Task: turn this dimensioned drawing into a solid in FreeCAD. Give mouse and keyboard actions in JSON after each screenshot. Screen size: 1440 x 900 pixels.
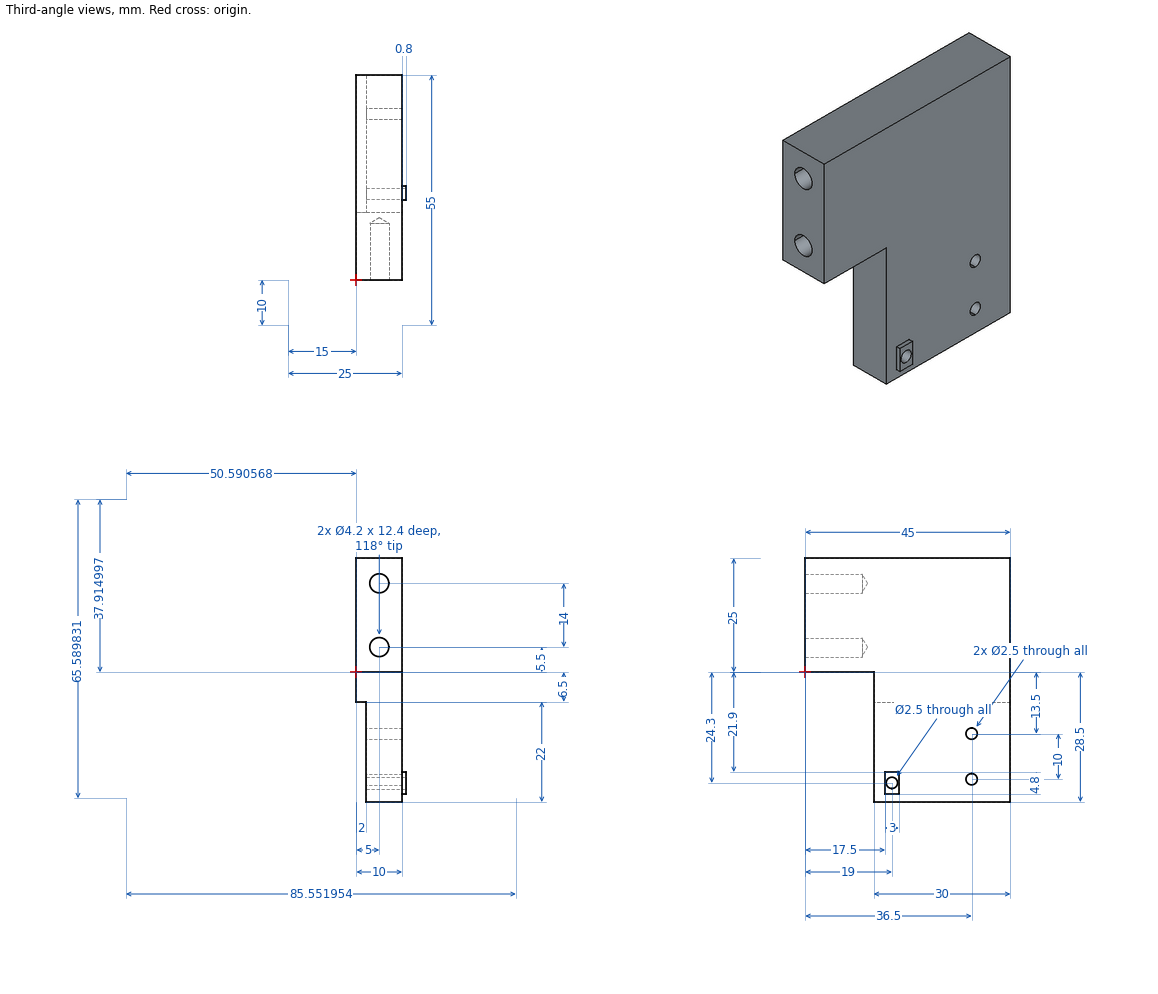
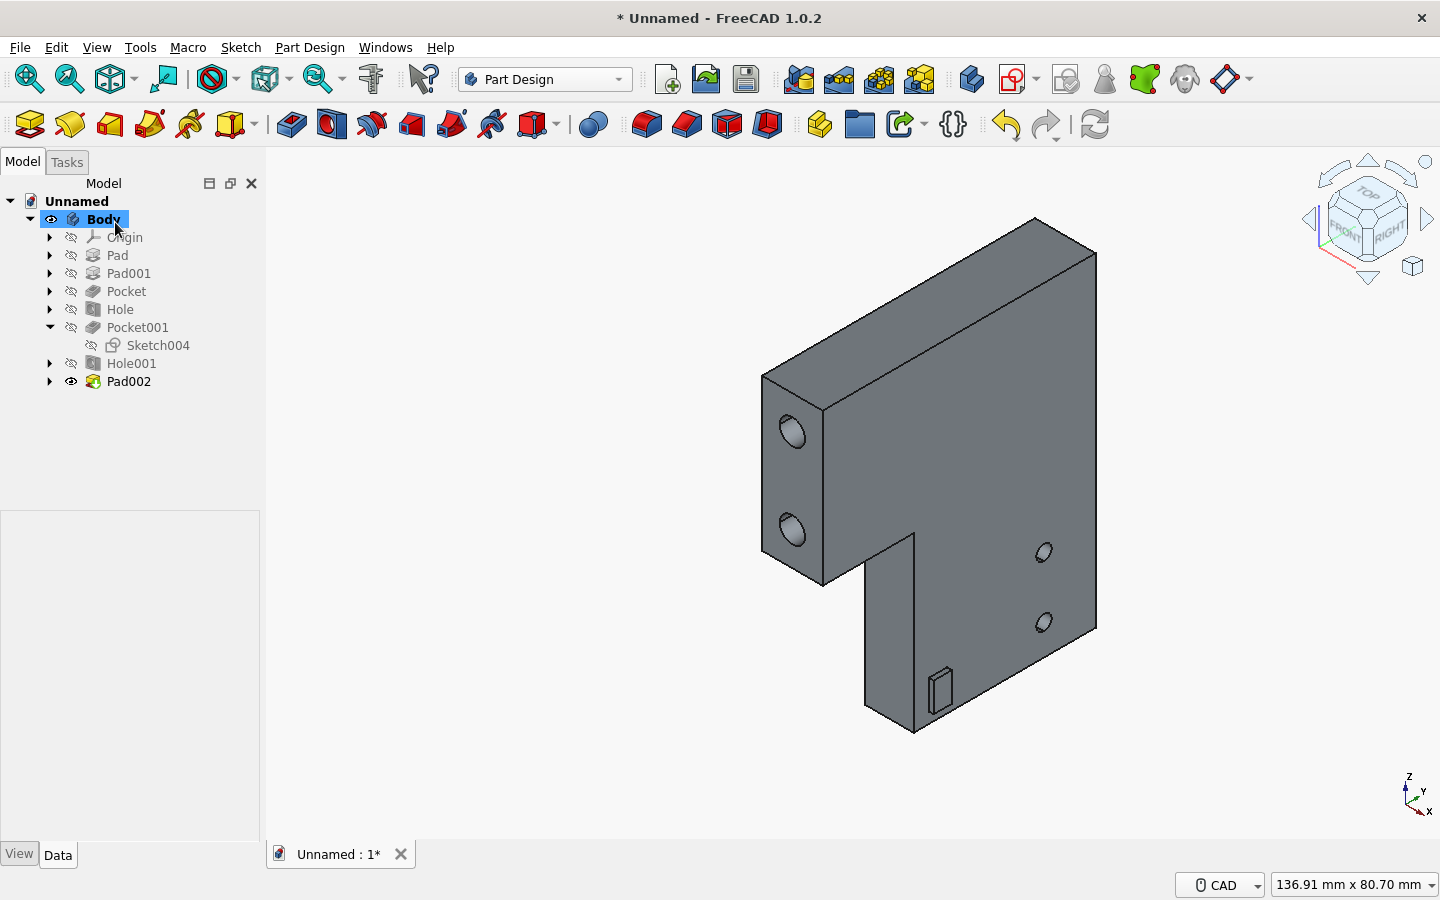
{"action": "left_click", "coordinate": [1012, 80]}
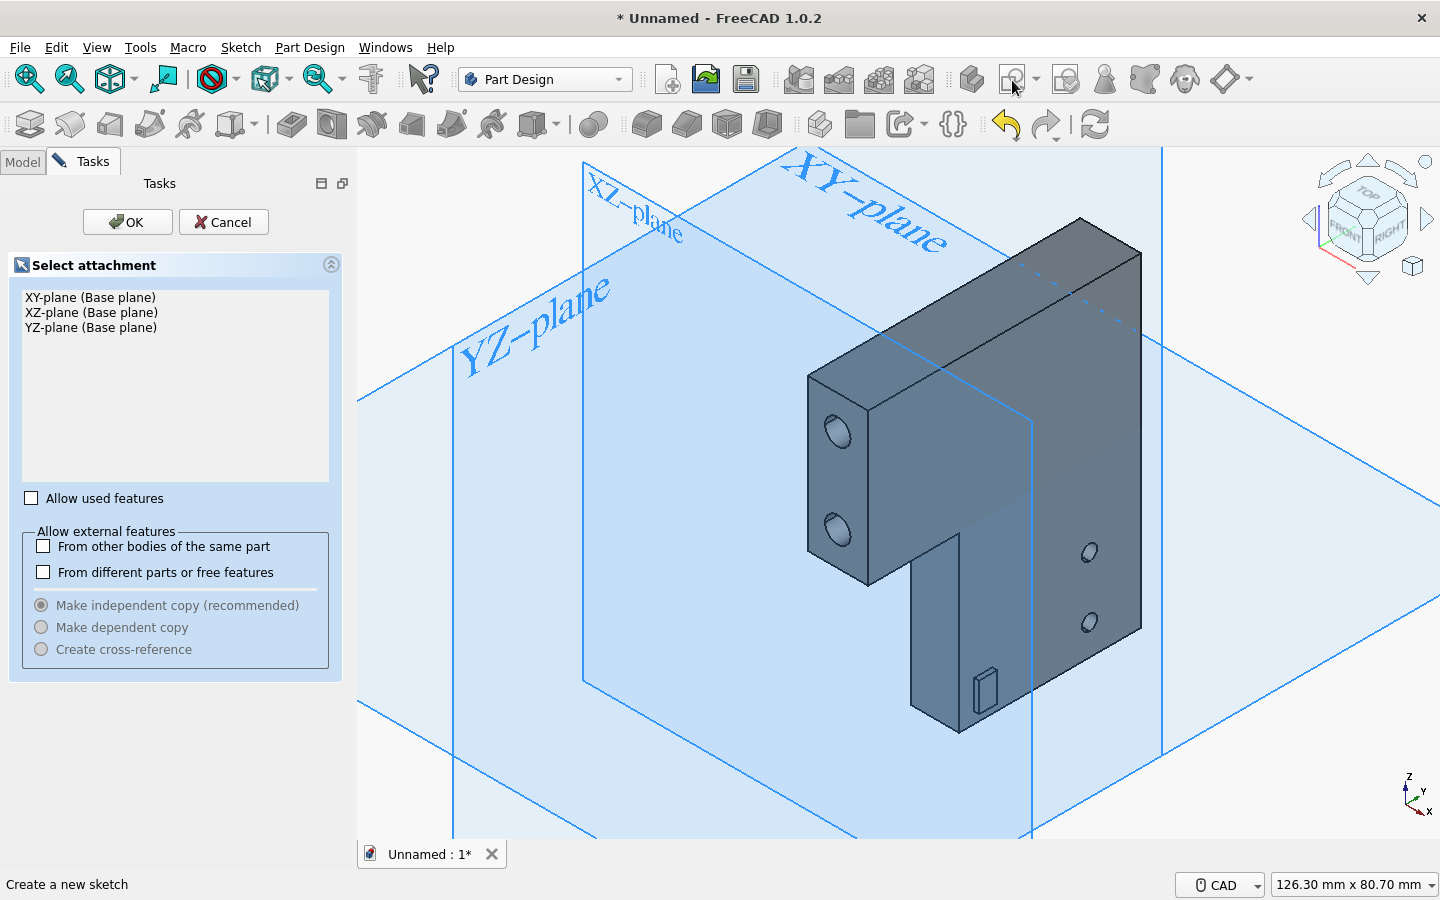
{"action": "left_click", "coordinate": [82, 328]}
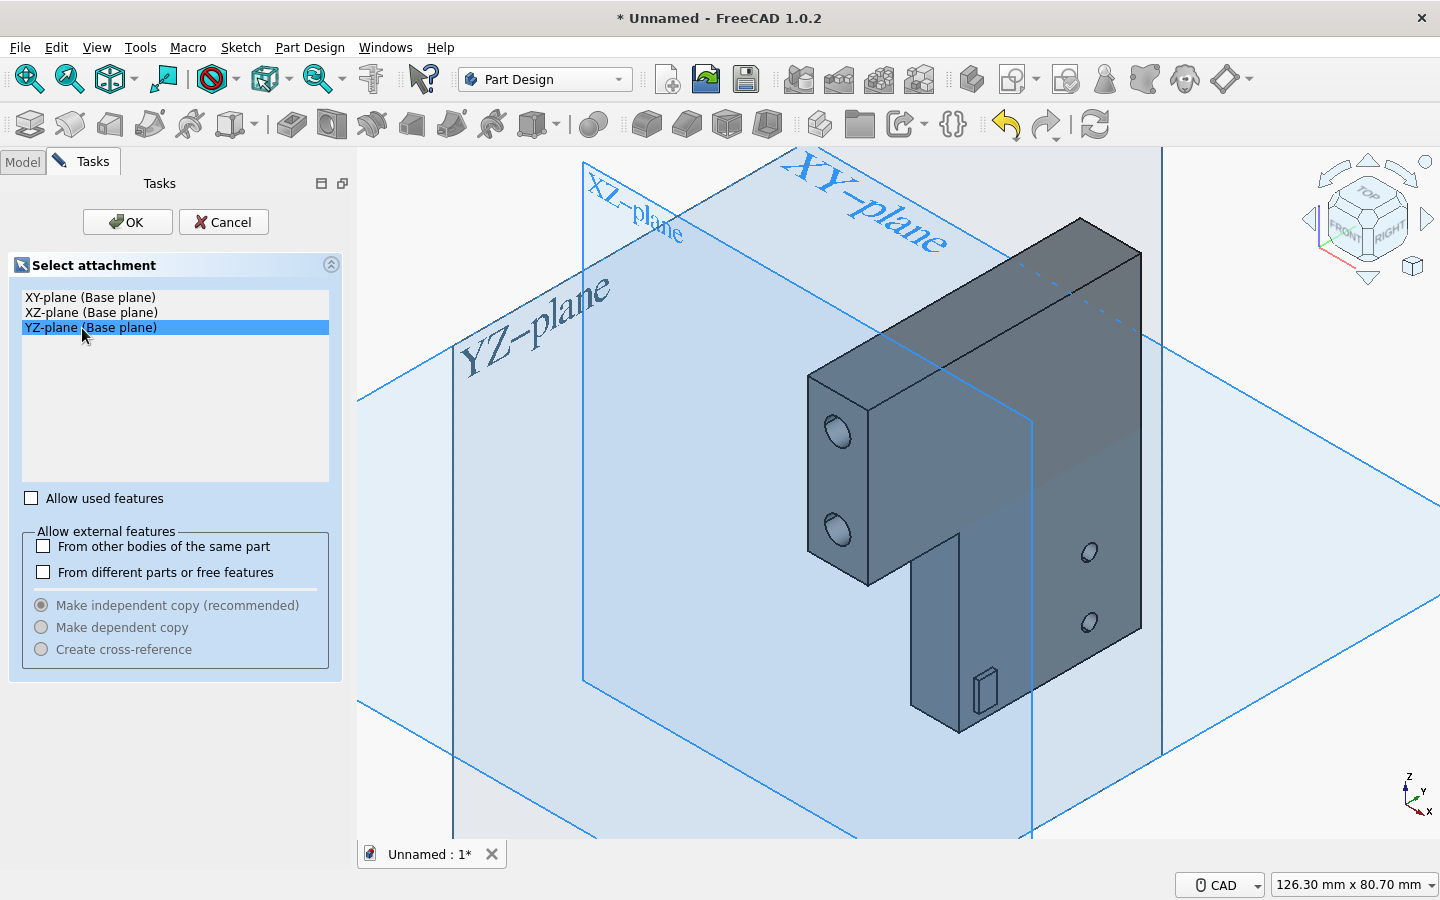
{"action": "left_click", "coordinate": [128, 222]}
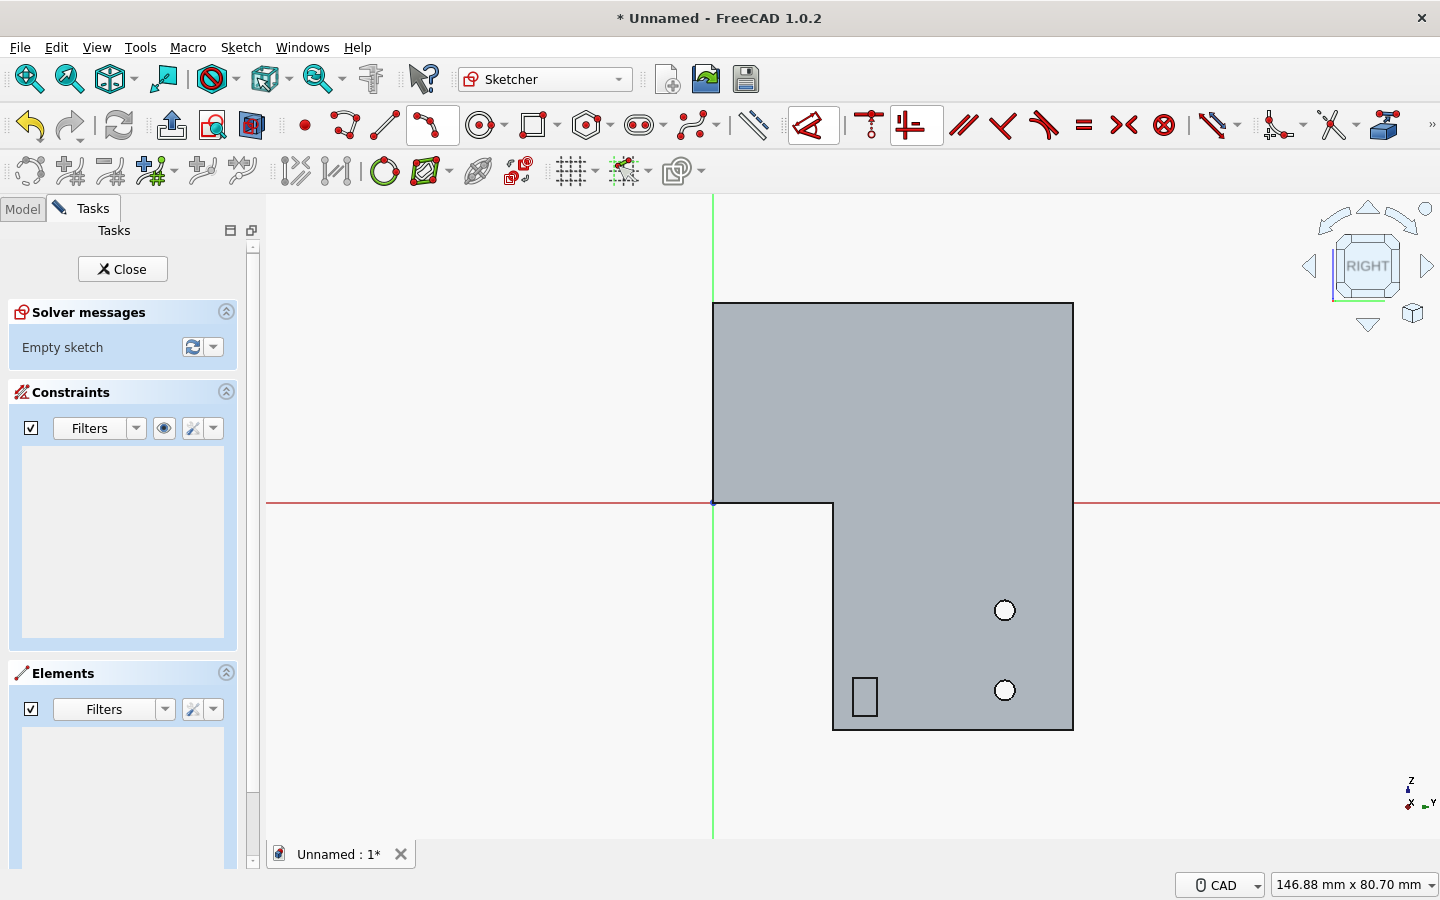
{"action": "left_click", "coordinate": [252, 126]}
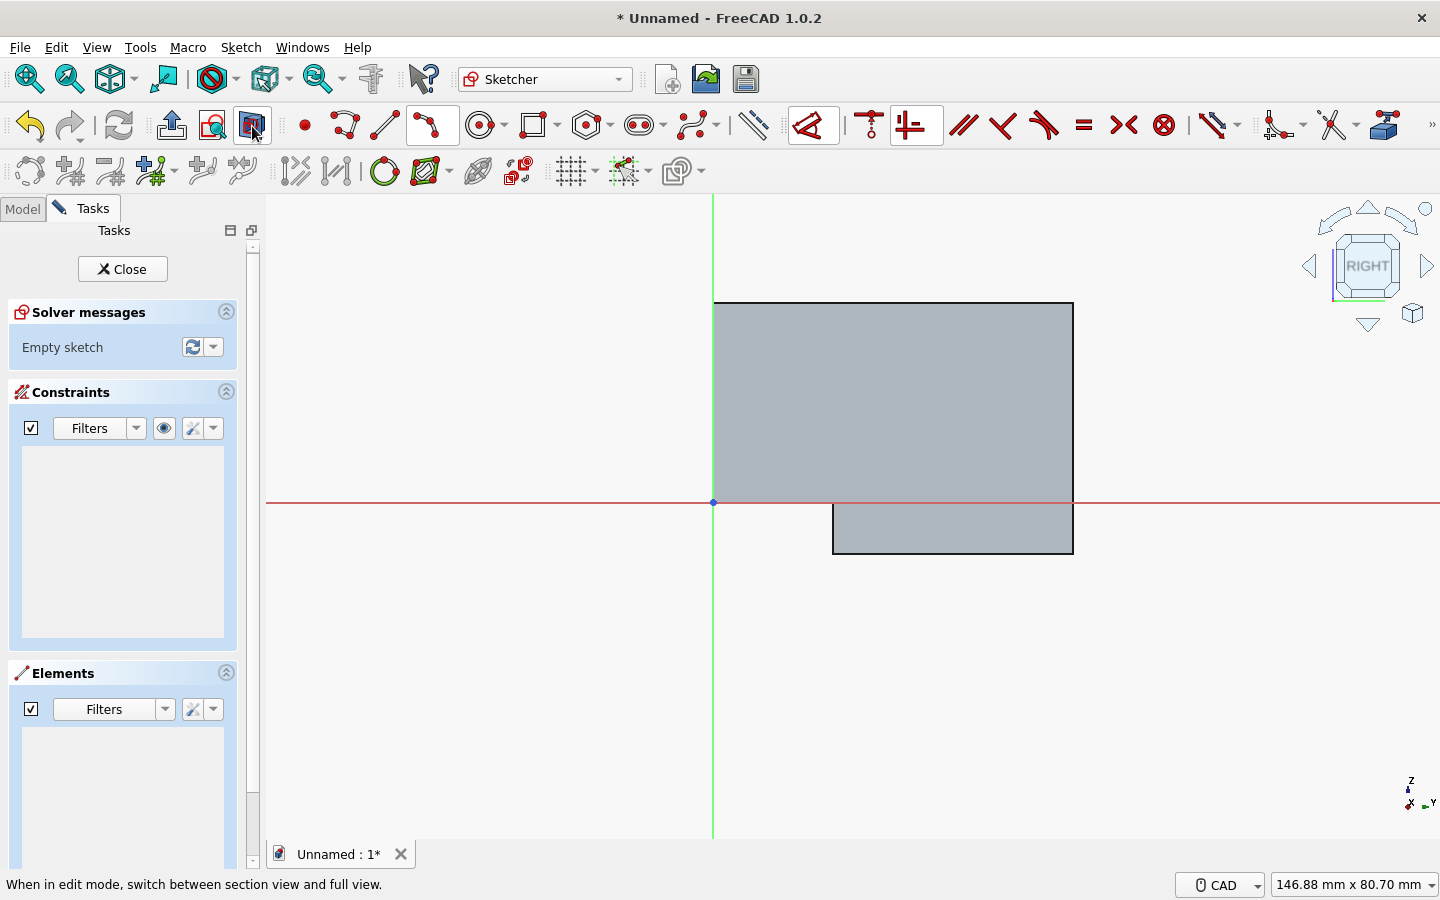
{"action": "scroll", "coordinate": [869, 706], "scroll_direction": "up", "scroll_amount": 15}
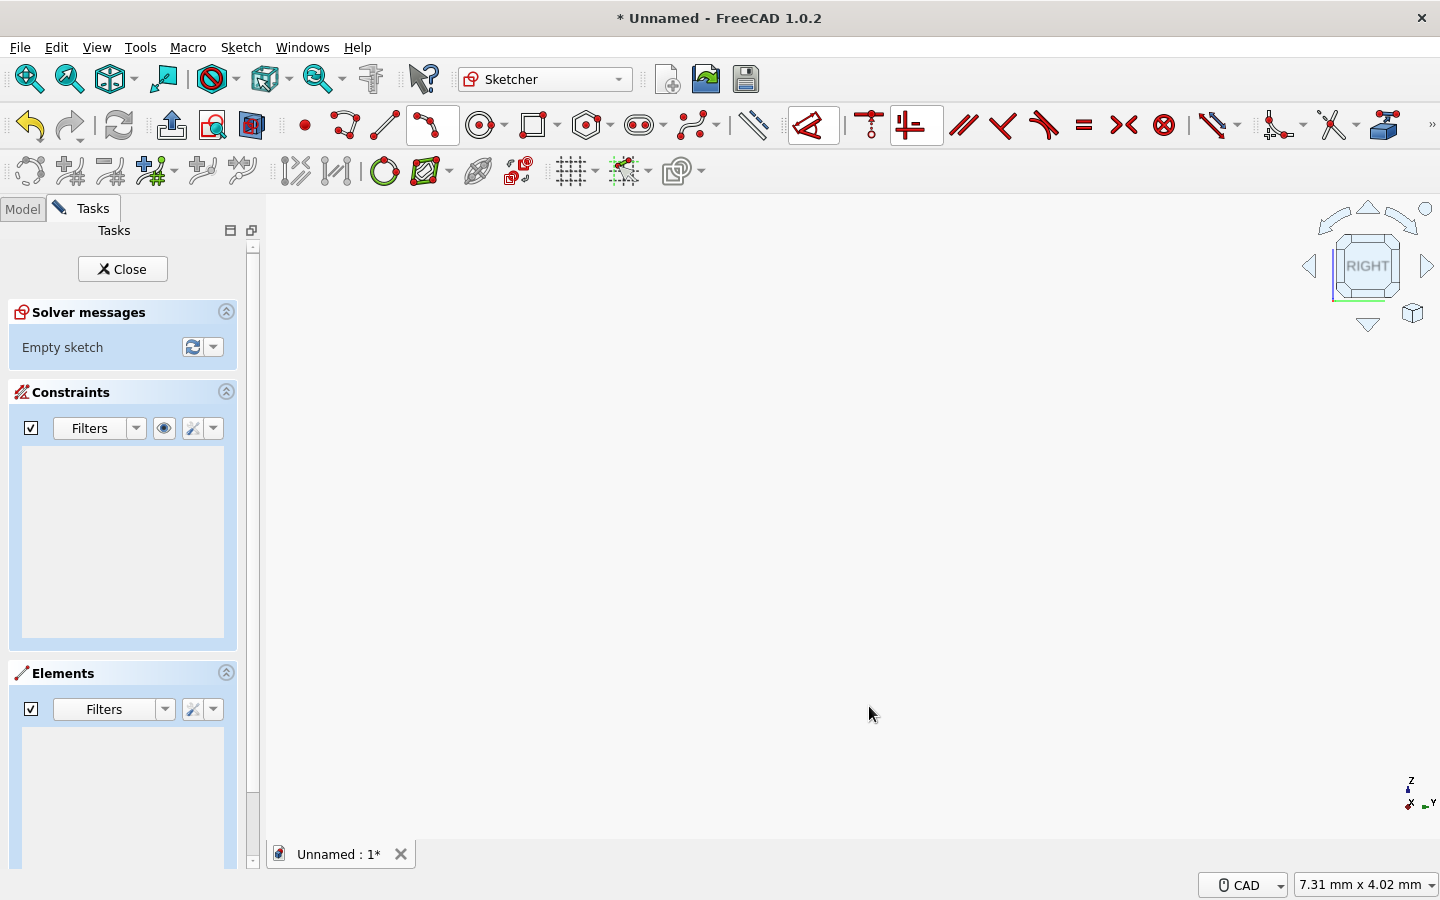
{"action": "left_click", "coordinate": [480, 126]}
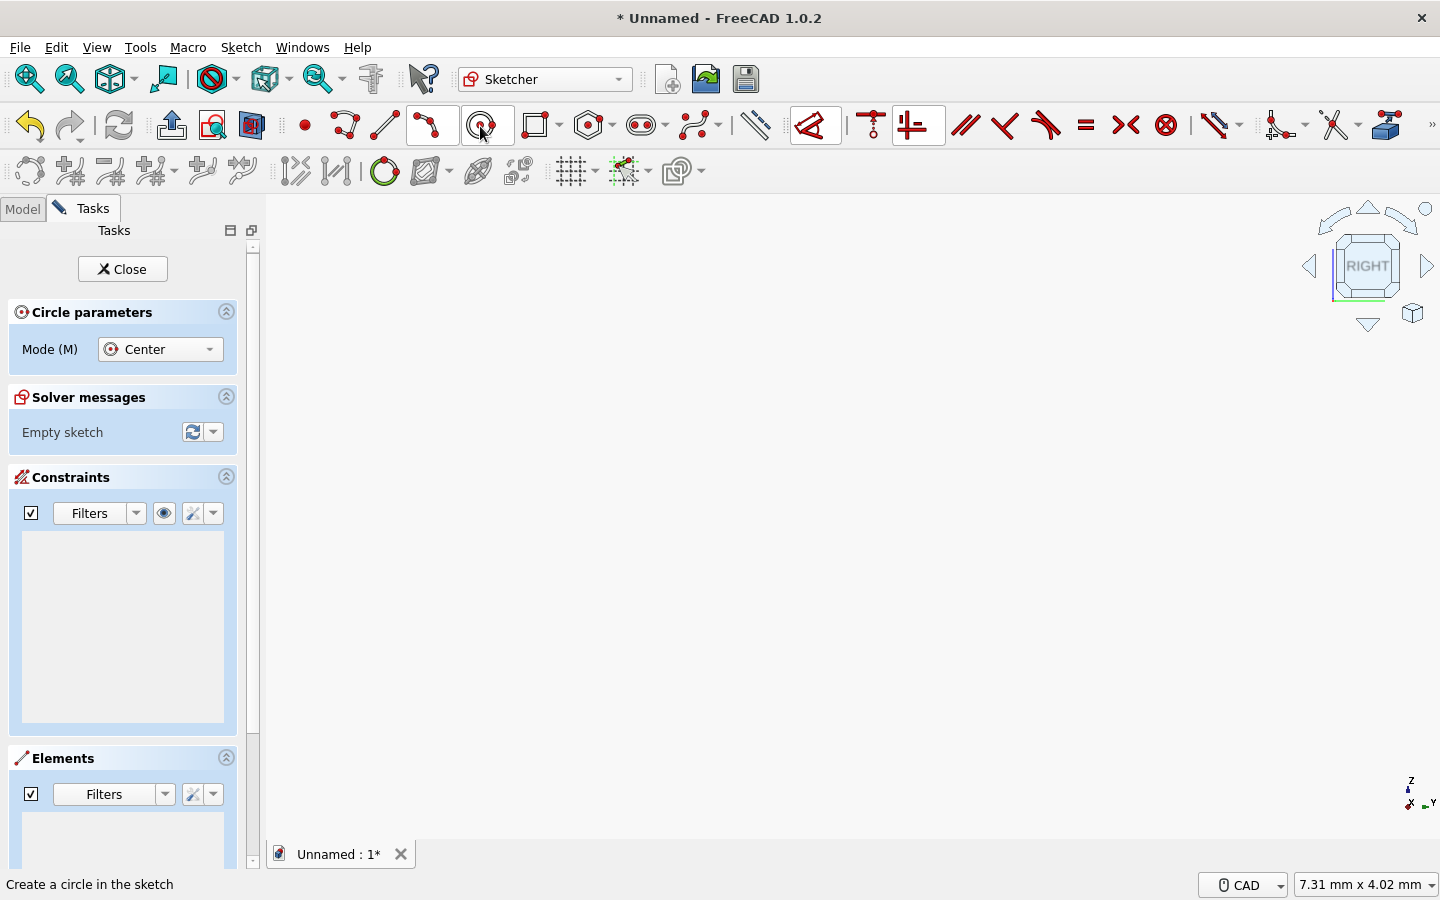
{"action": "left_click", "coordinate": [779, 505]}
{"action": "left_click", "coordinate": [921, 363]}
{"action": "key", "text": "Escape"}